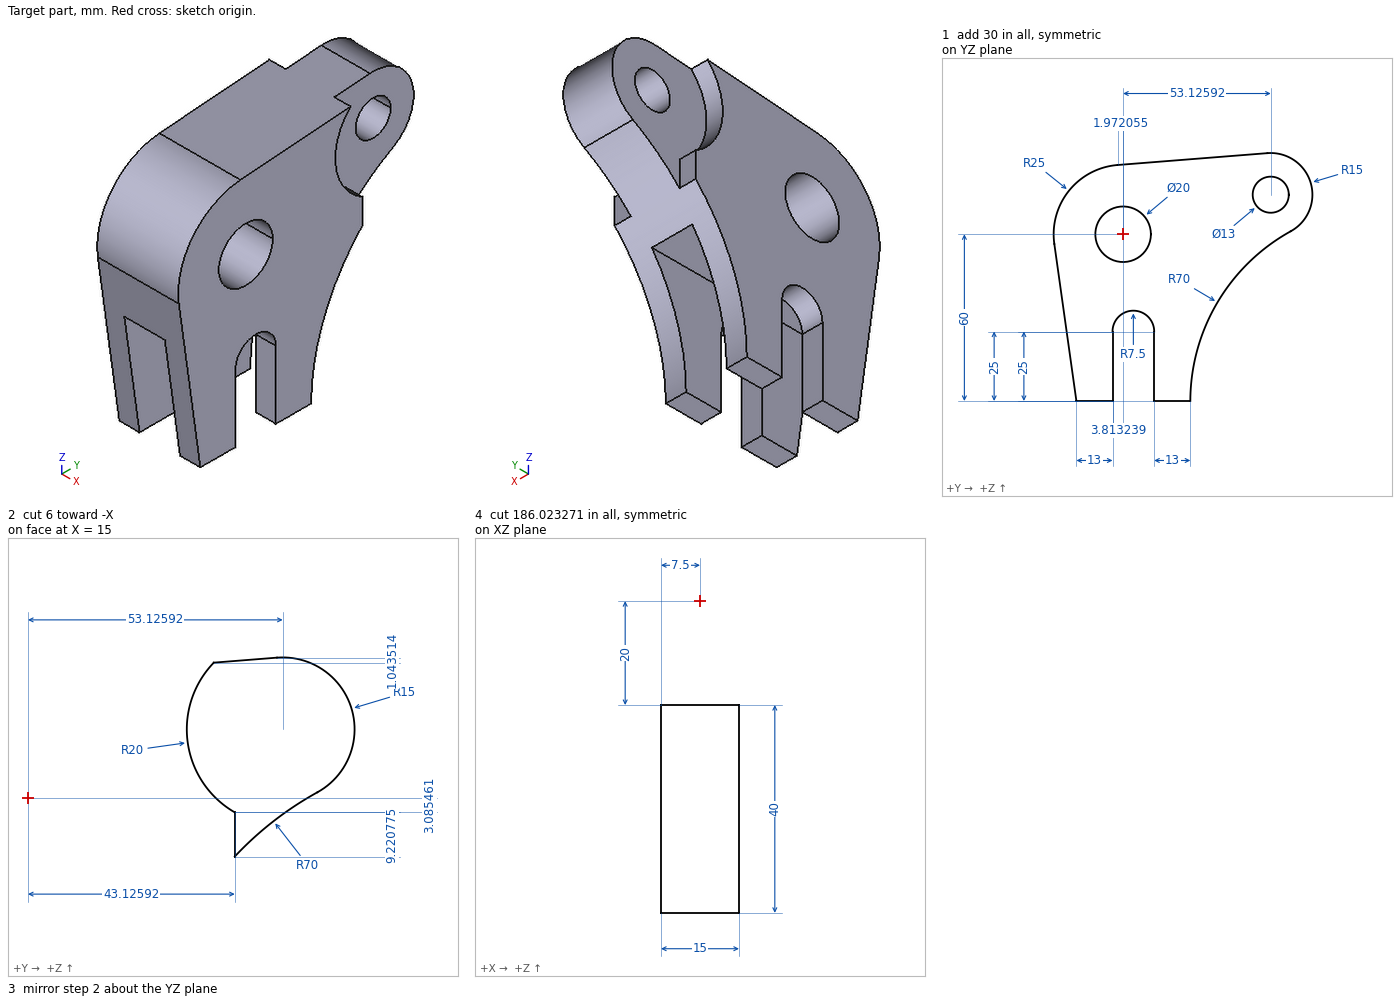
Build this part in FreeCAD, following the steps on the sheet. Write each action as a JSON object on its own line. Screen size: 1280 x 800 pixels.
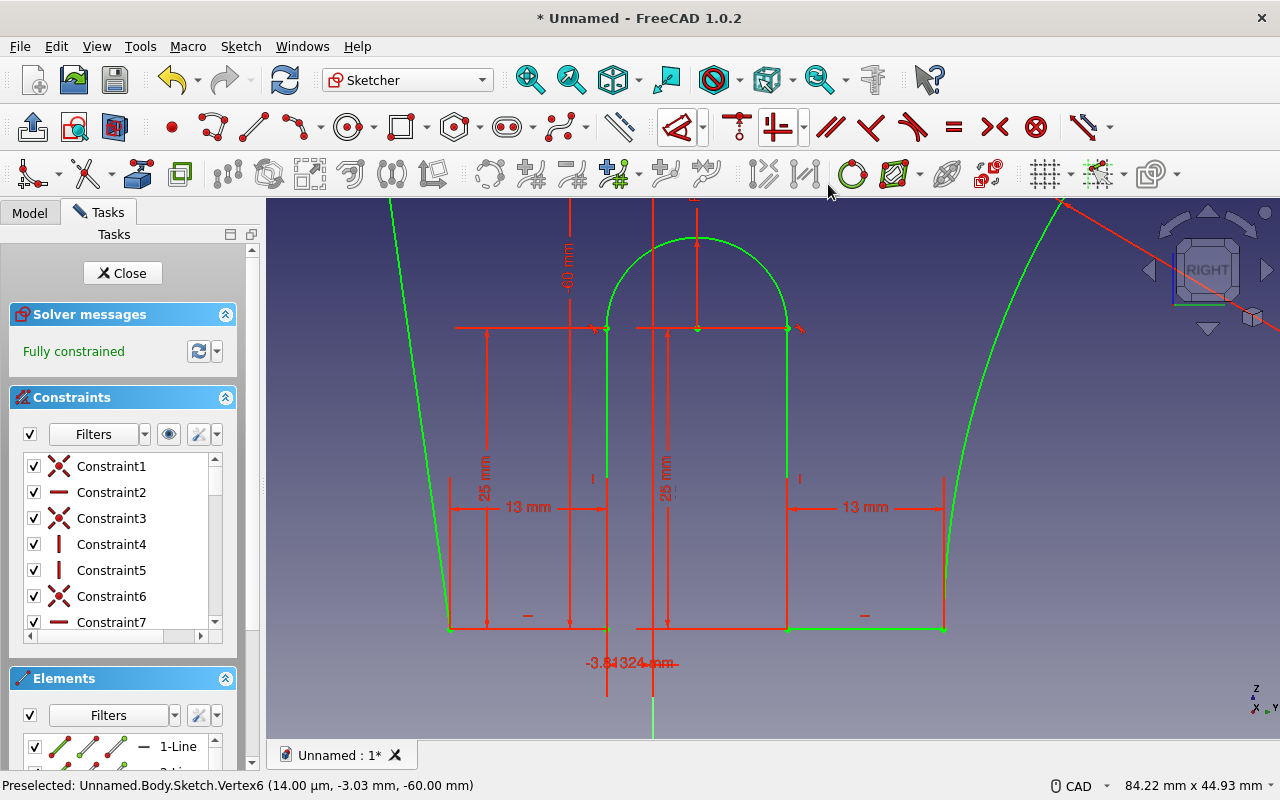
{"action": "left_click", "coordinate": [123, 273]}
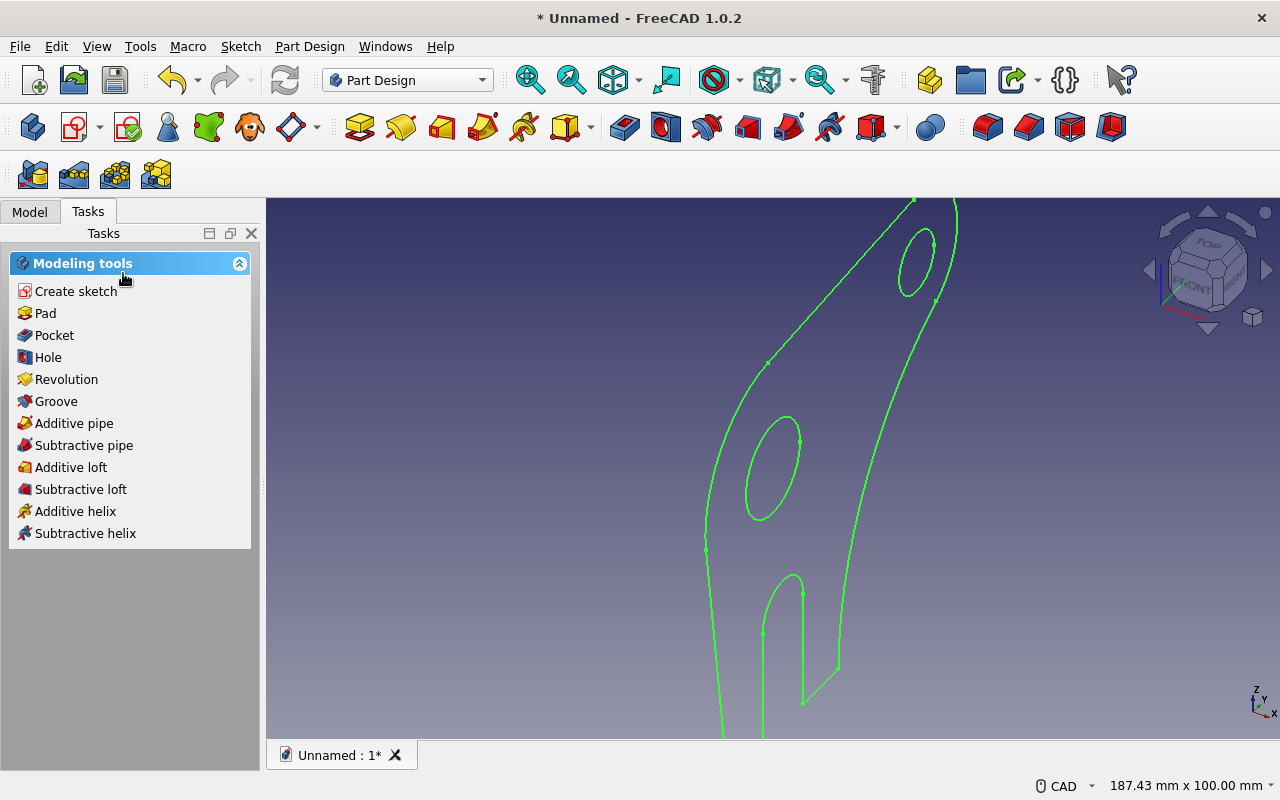
{"action": "left_click", "coordinate": [360, 128]}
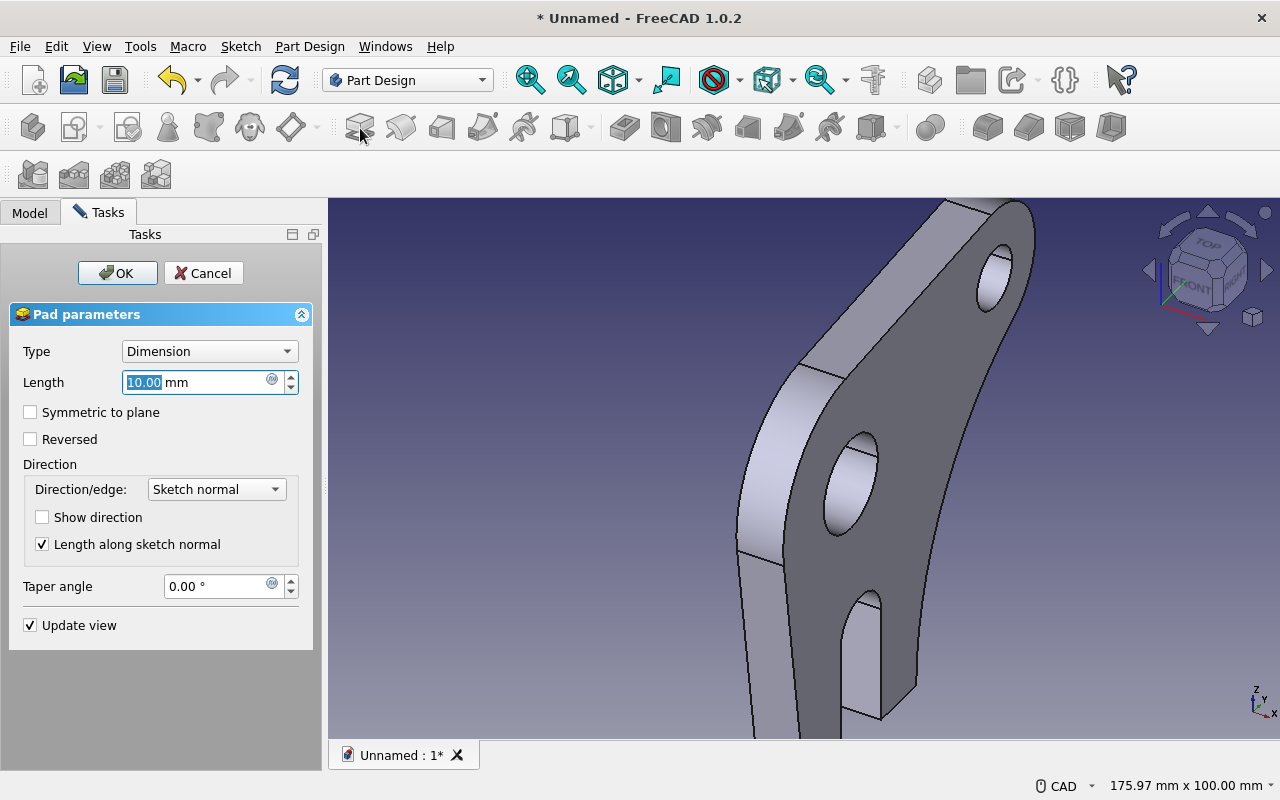
{"action": "type", "text": "30"}
{"action": "key", "text": "Tab"}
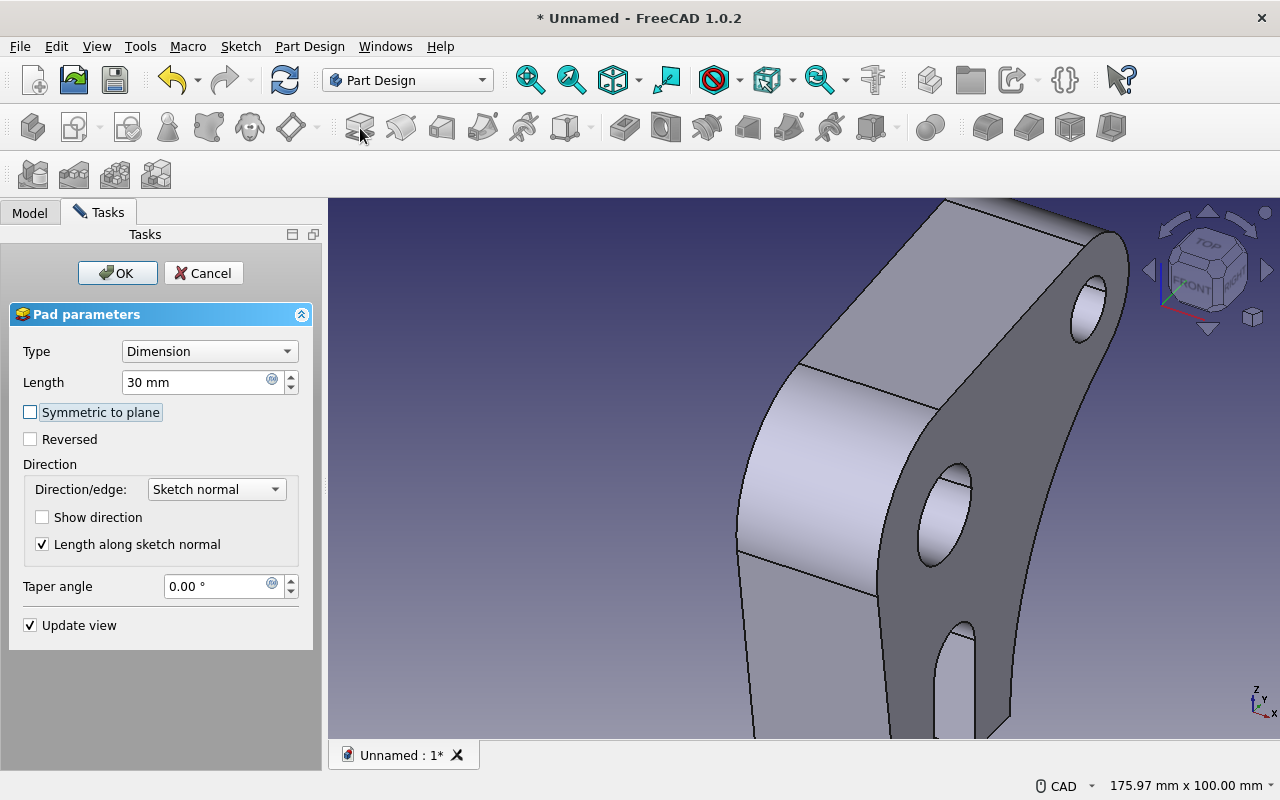
{"action": "left_click", "coordinate": [31, 412]}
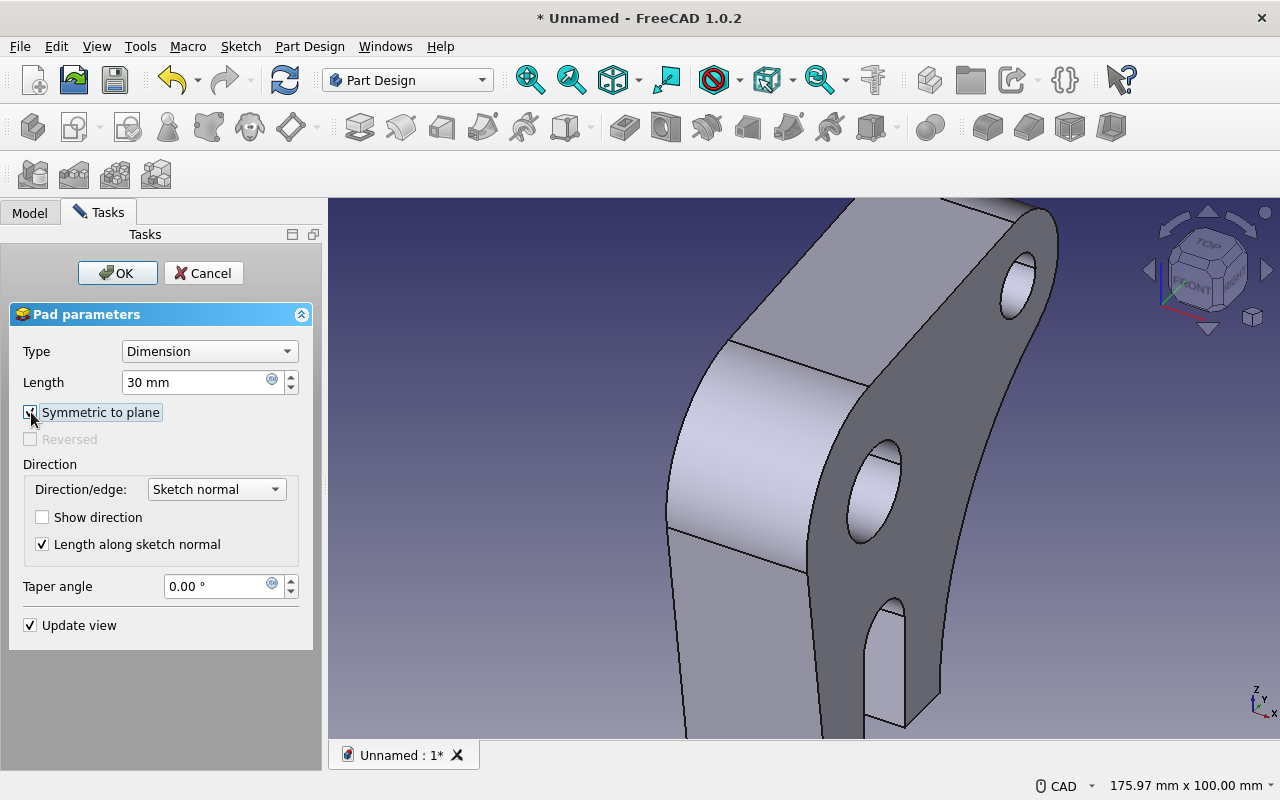
{"action": "left_click", "coordinate": [118, 273]}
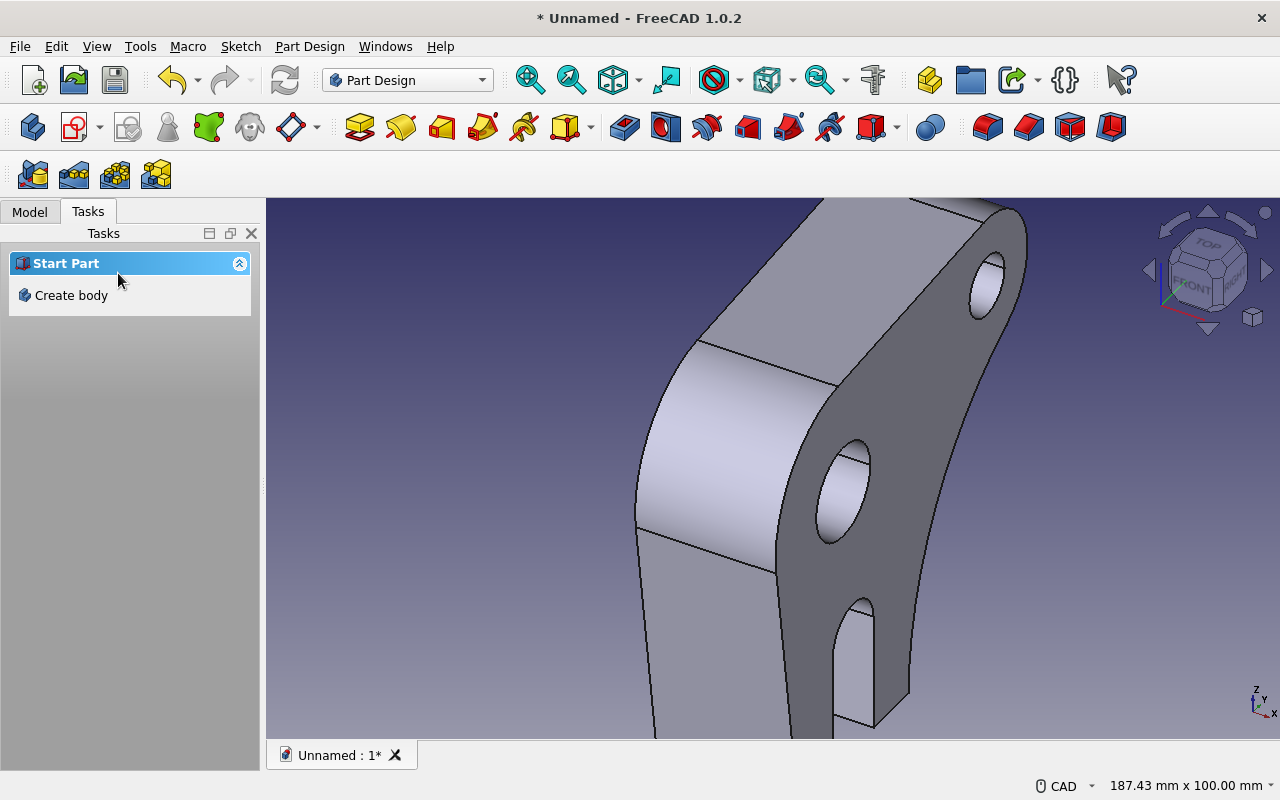
{"action": "left_click", "coordinate": [531, 80]}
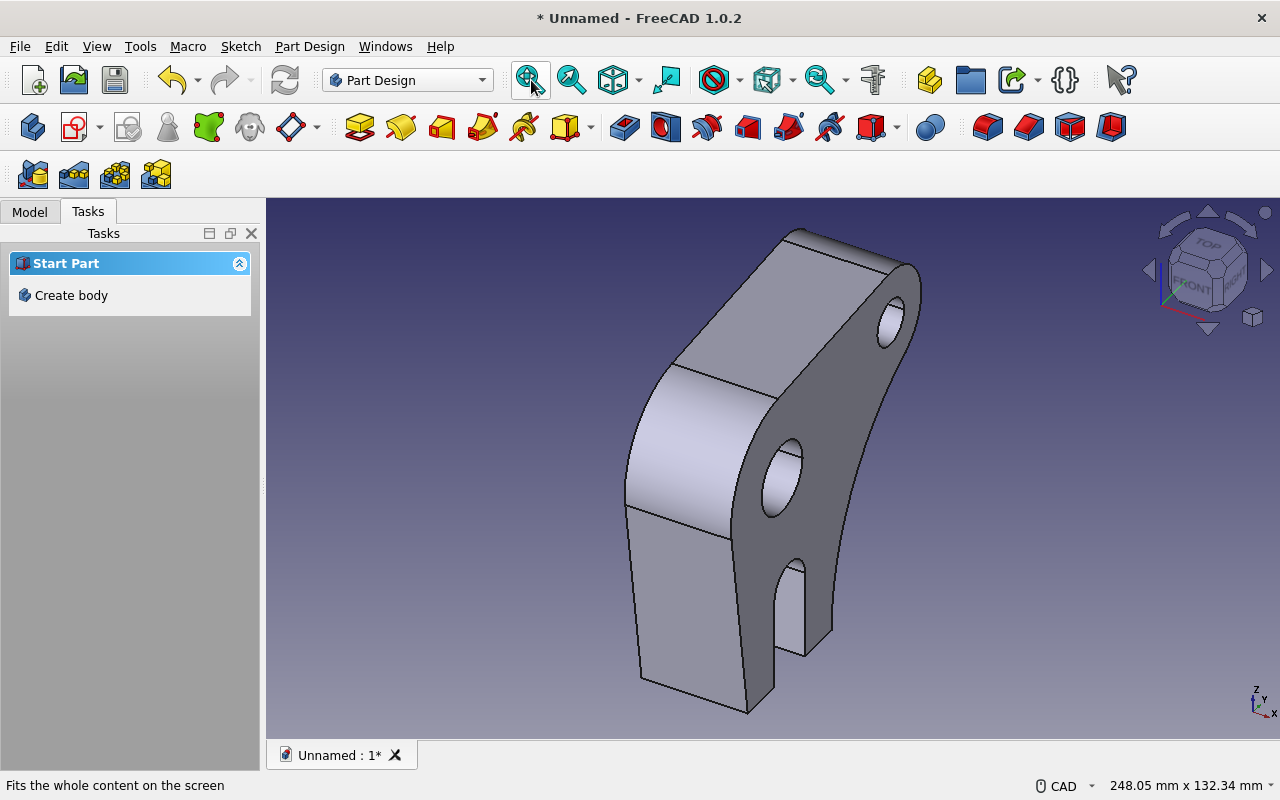
{"action": "left_click", "coordinate": [826, 485]}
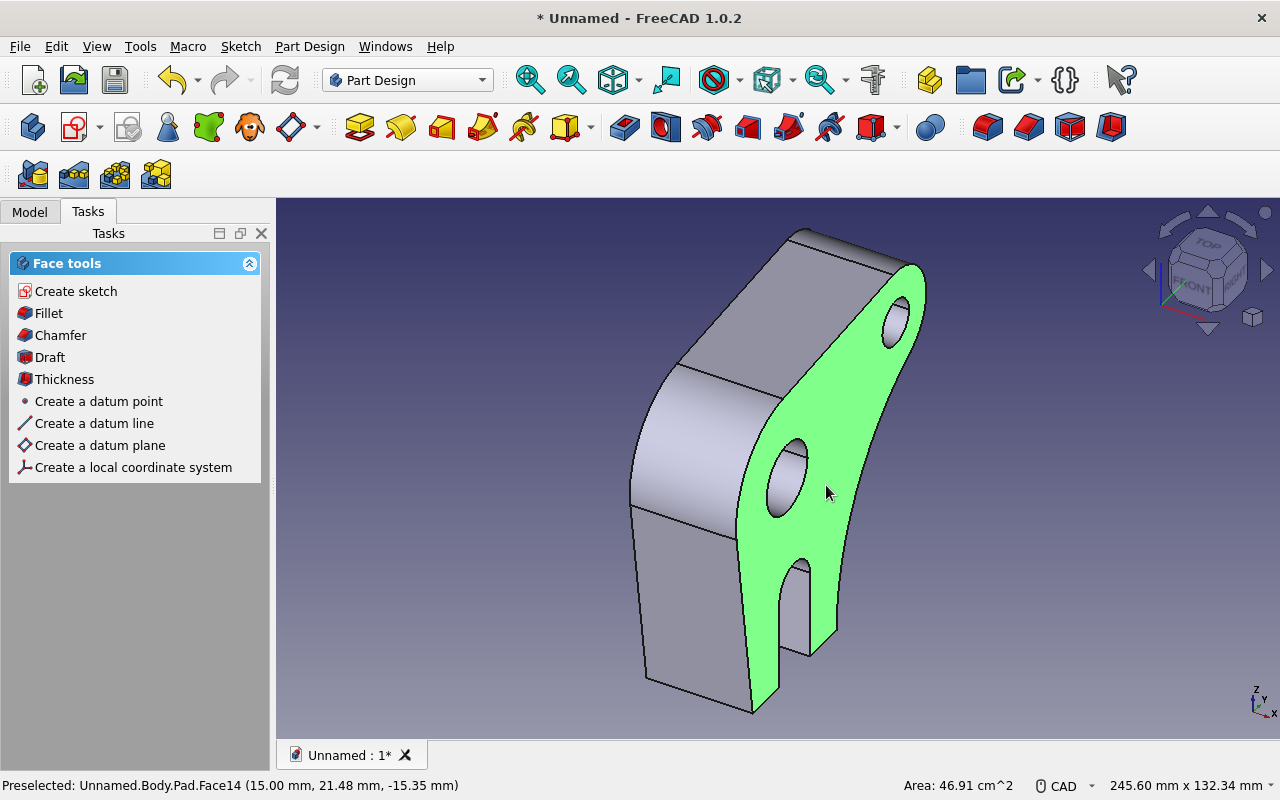
{"action": "left_click", "coordinate": [74, 128]}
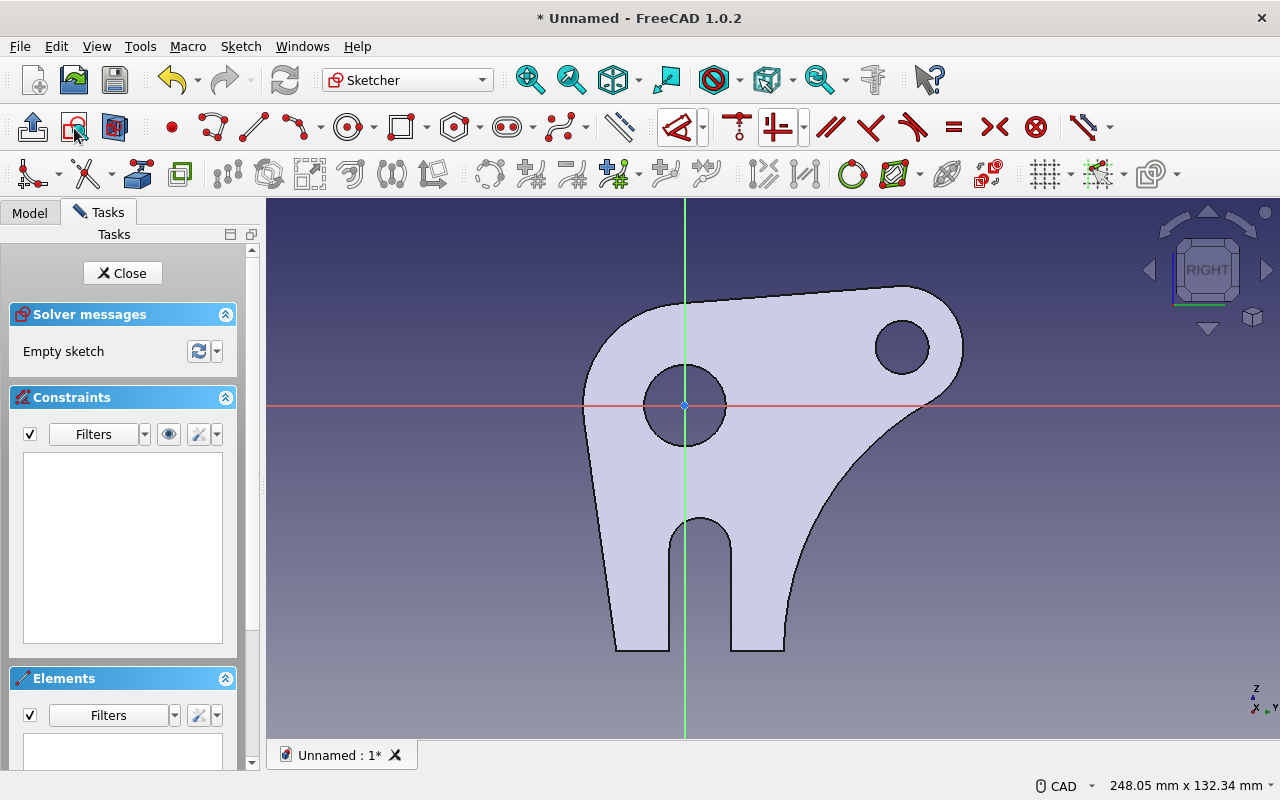
{"action": "scroll", "coordinate": [920, 291], "scroll_direction": "up", "scroll_amount": 4}